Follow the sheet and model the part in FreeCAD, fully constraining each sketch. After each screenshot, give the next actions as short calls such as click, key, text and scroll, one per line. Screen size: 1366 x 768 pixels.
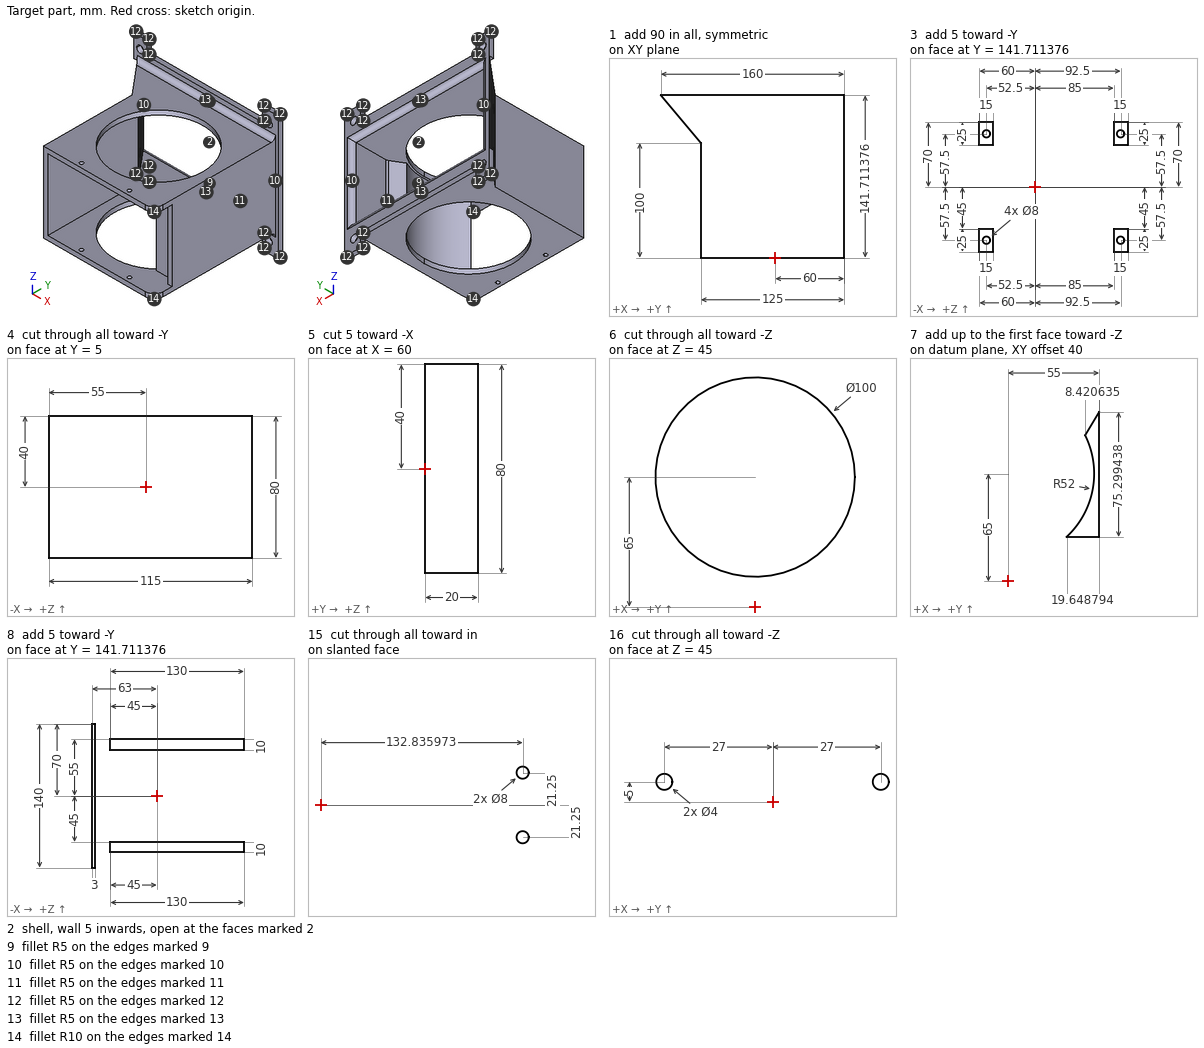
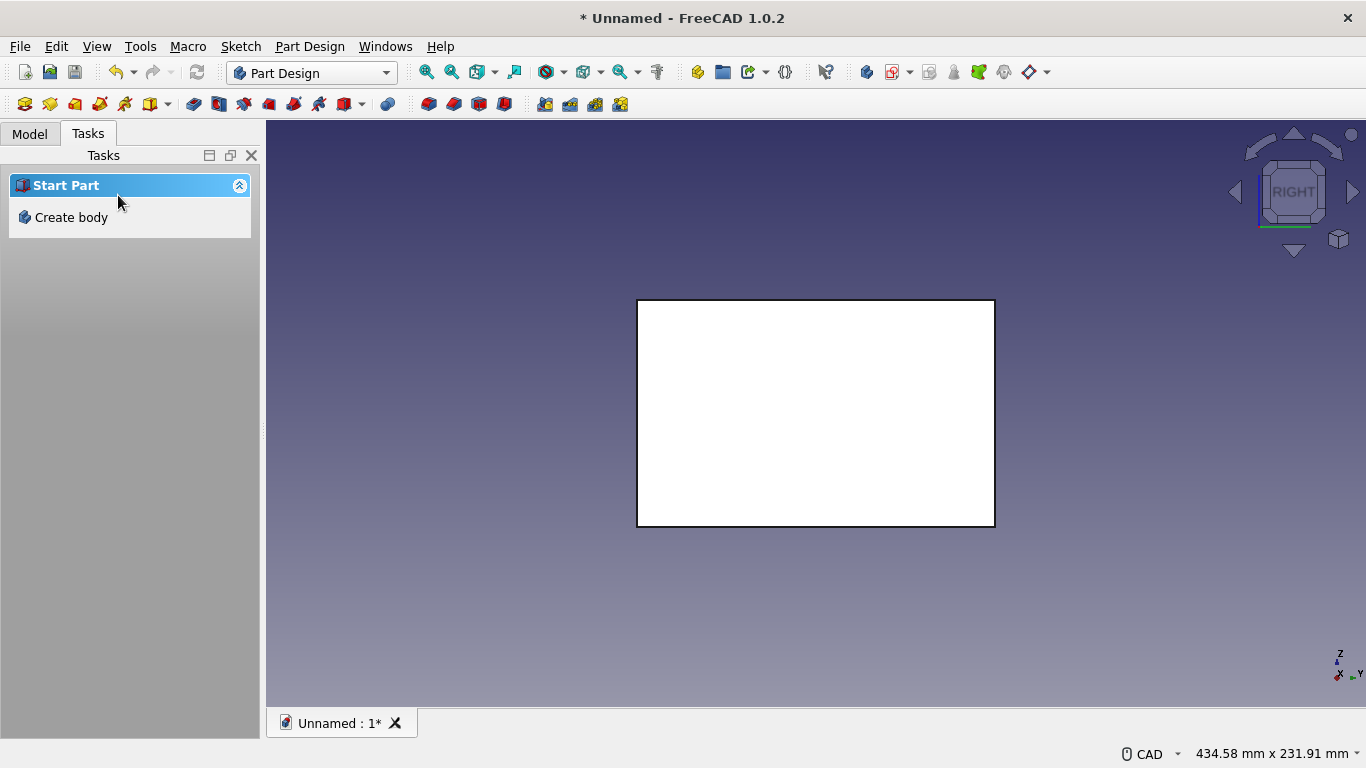
key(5)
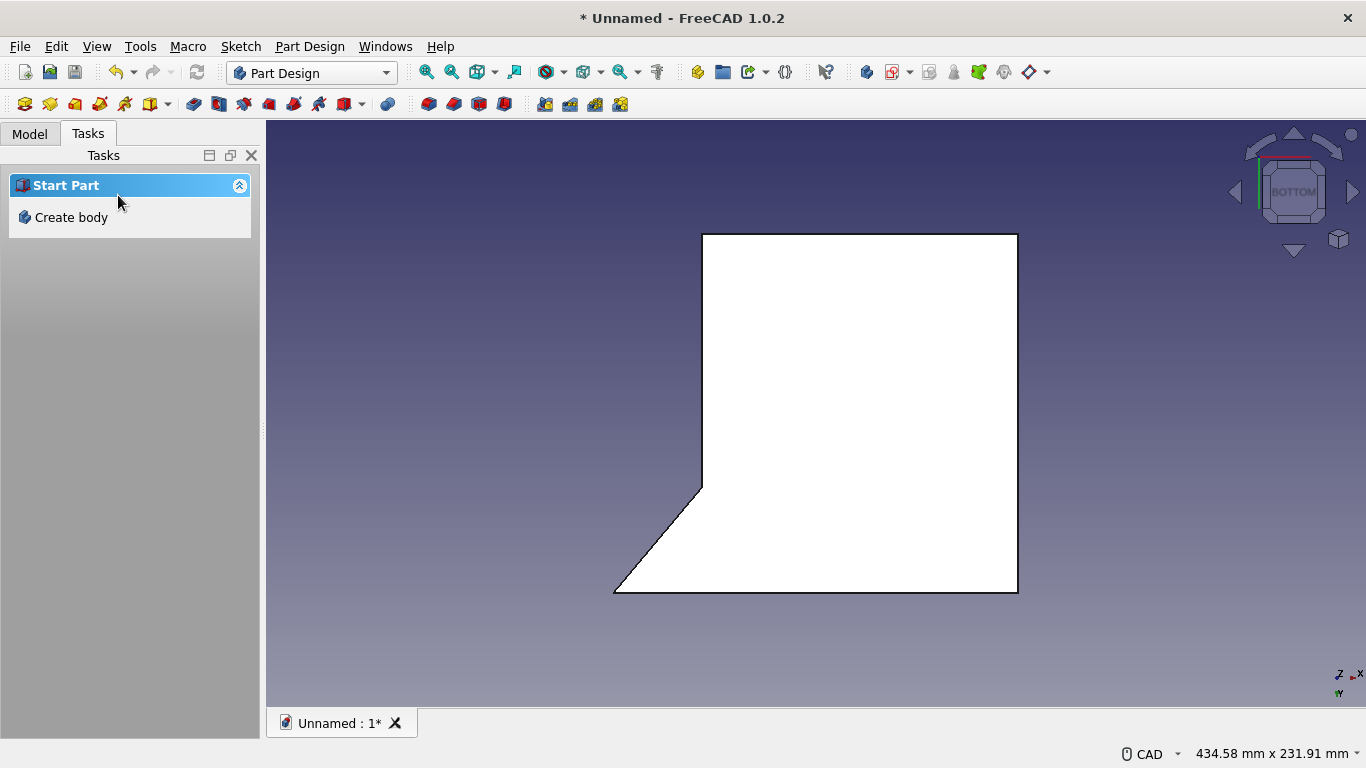
key(4)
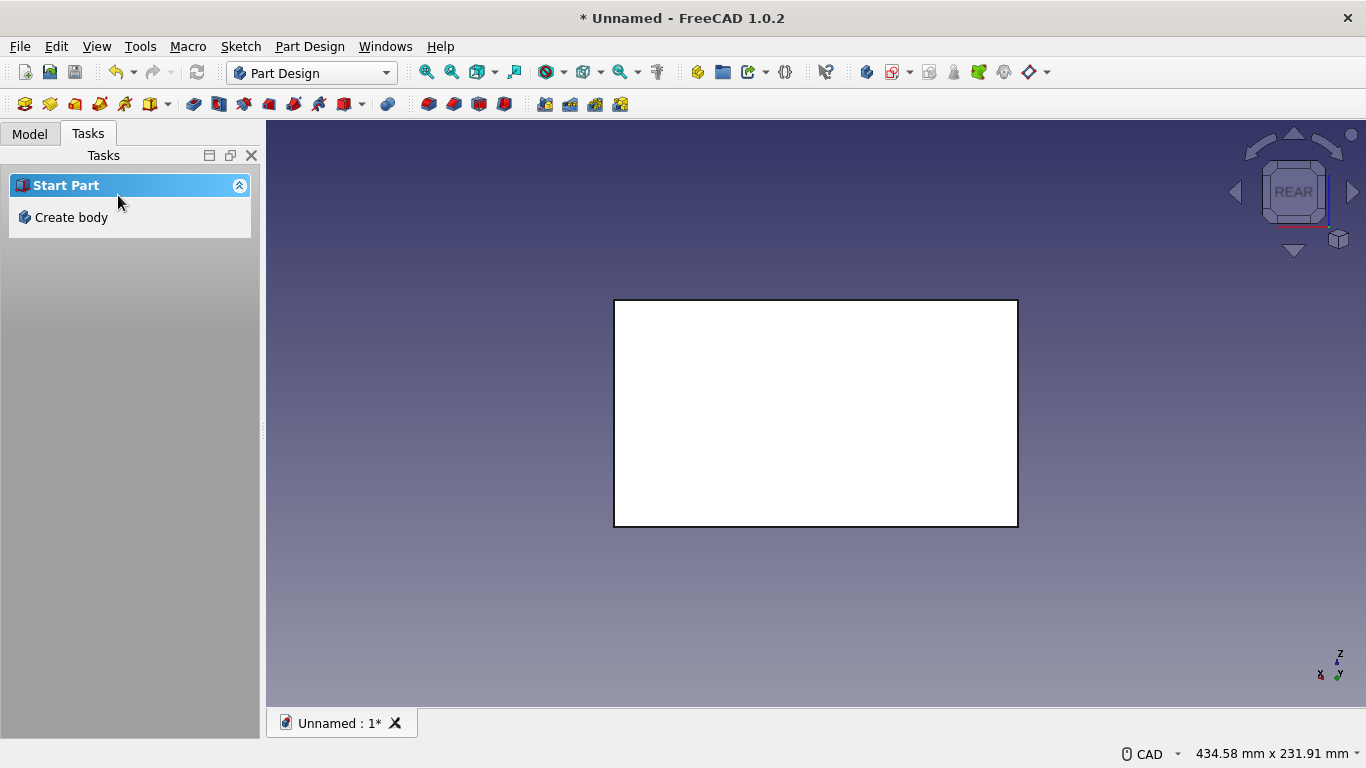
key(v)
key(f)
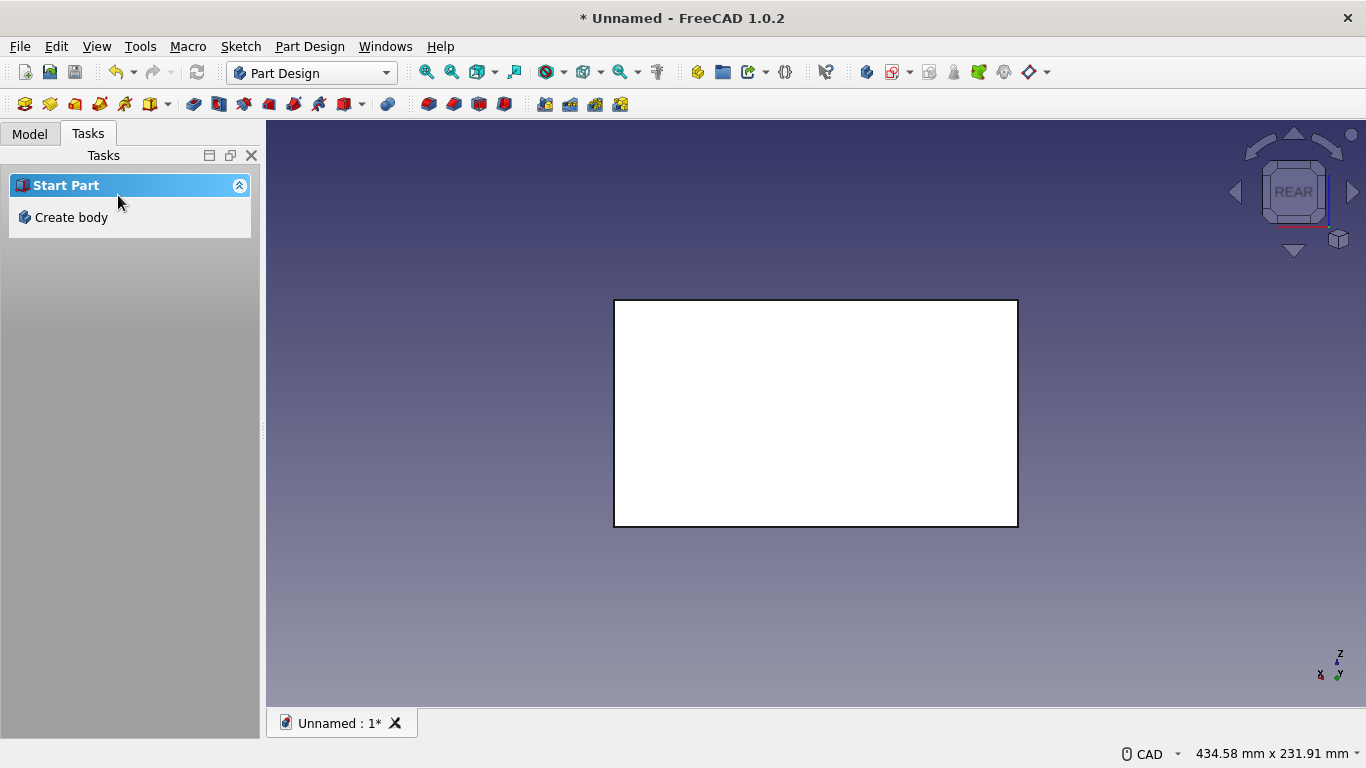
click(758, 413)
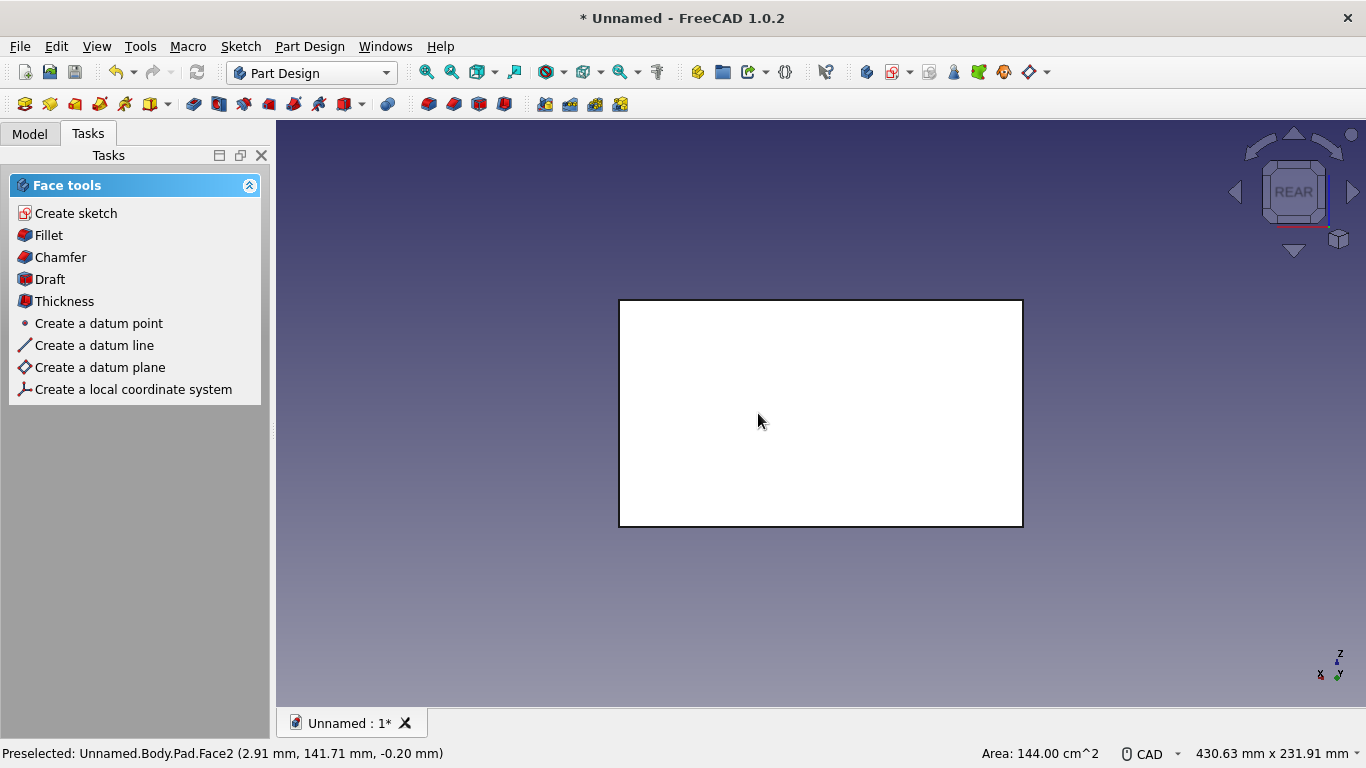
click(504, 104)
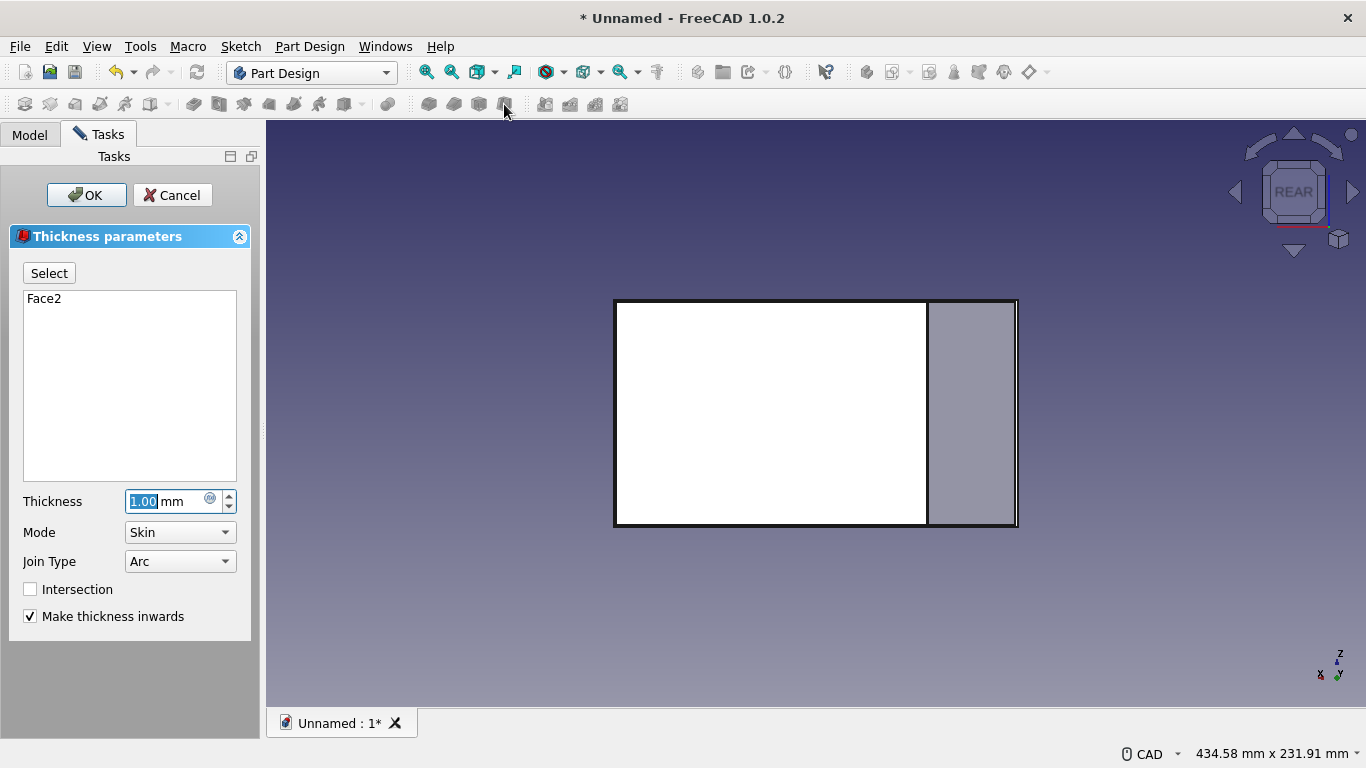
text(5)
key(Tab)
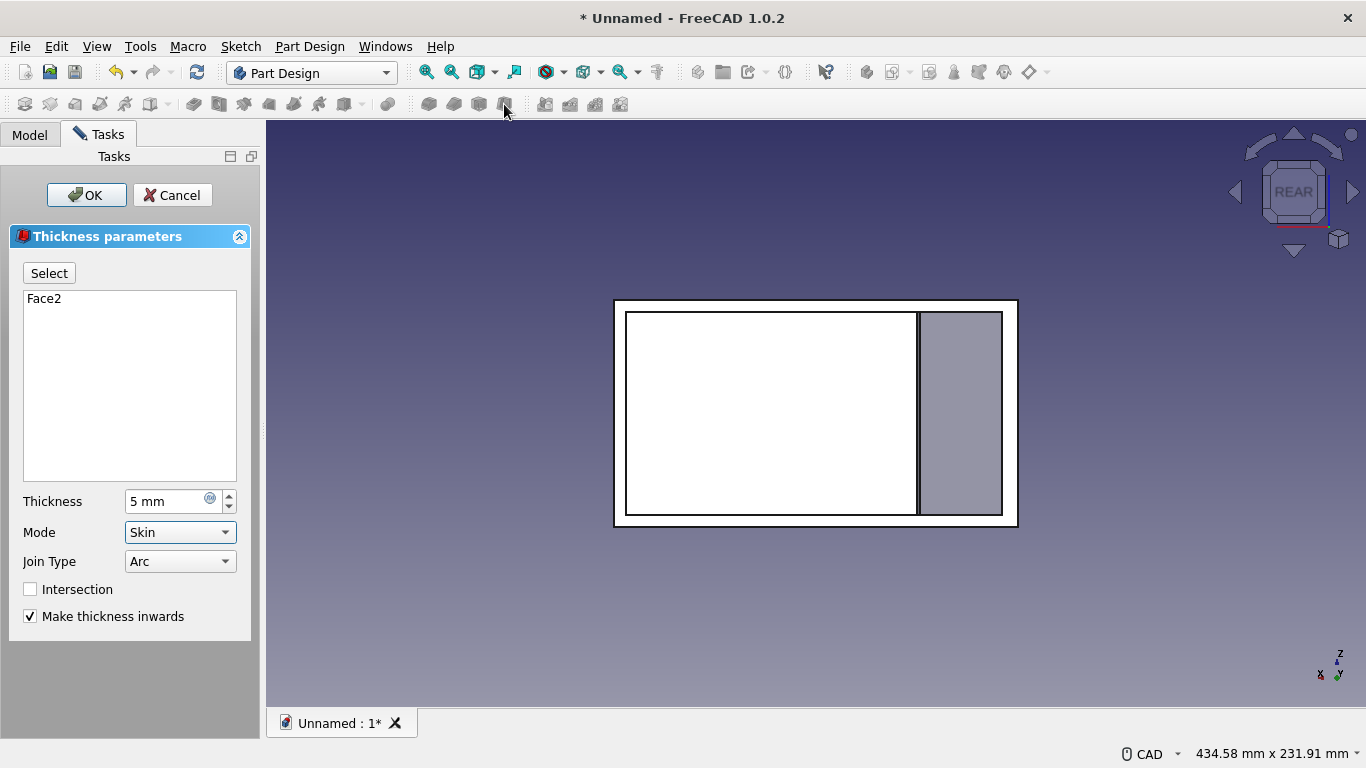
click(181, 562)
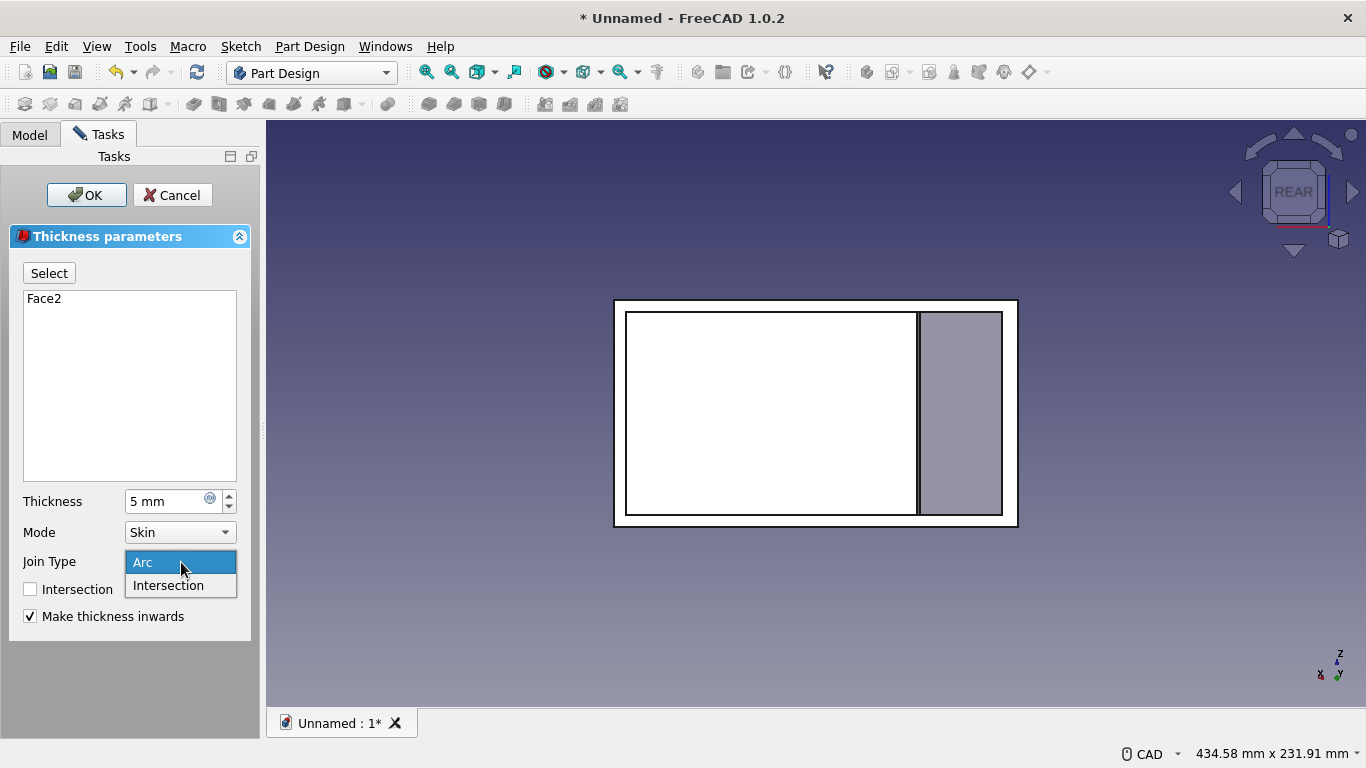
click(179, 586)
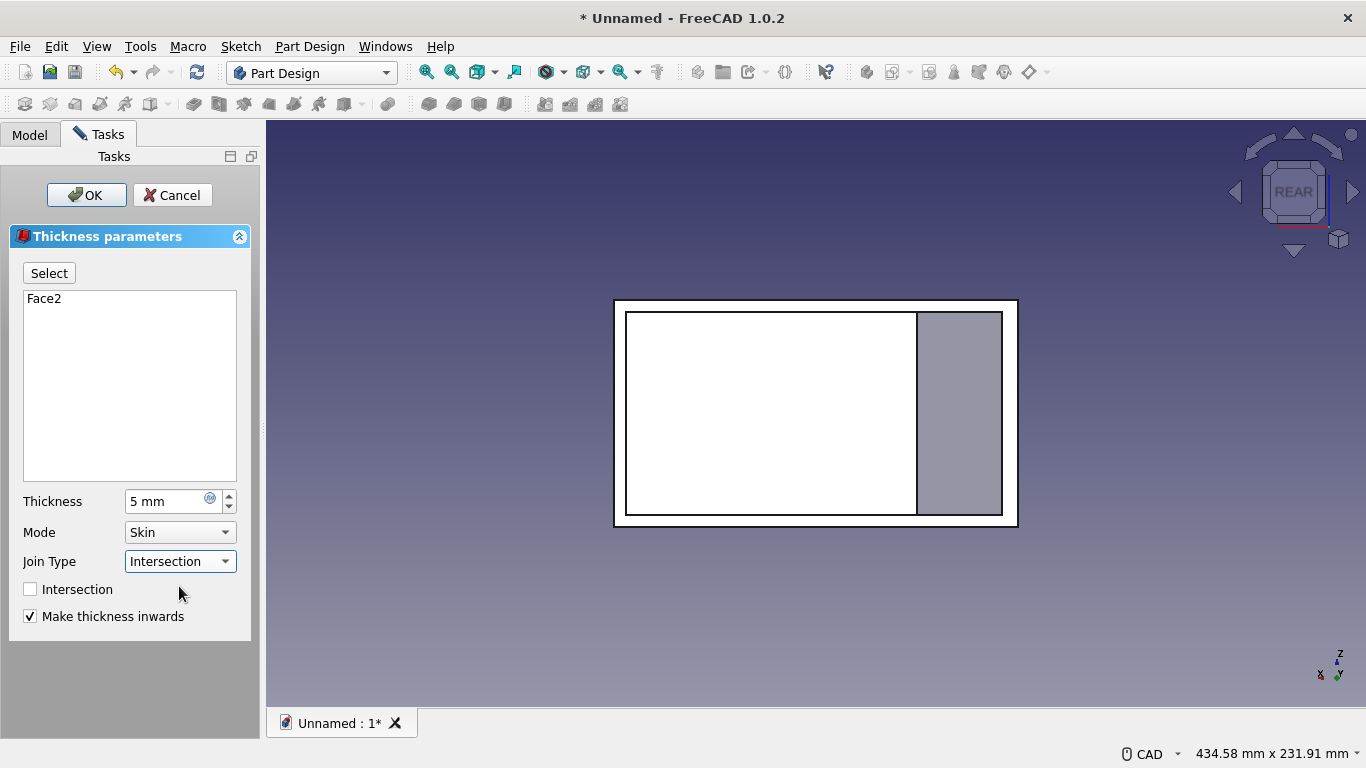
click(87, 195)